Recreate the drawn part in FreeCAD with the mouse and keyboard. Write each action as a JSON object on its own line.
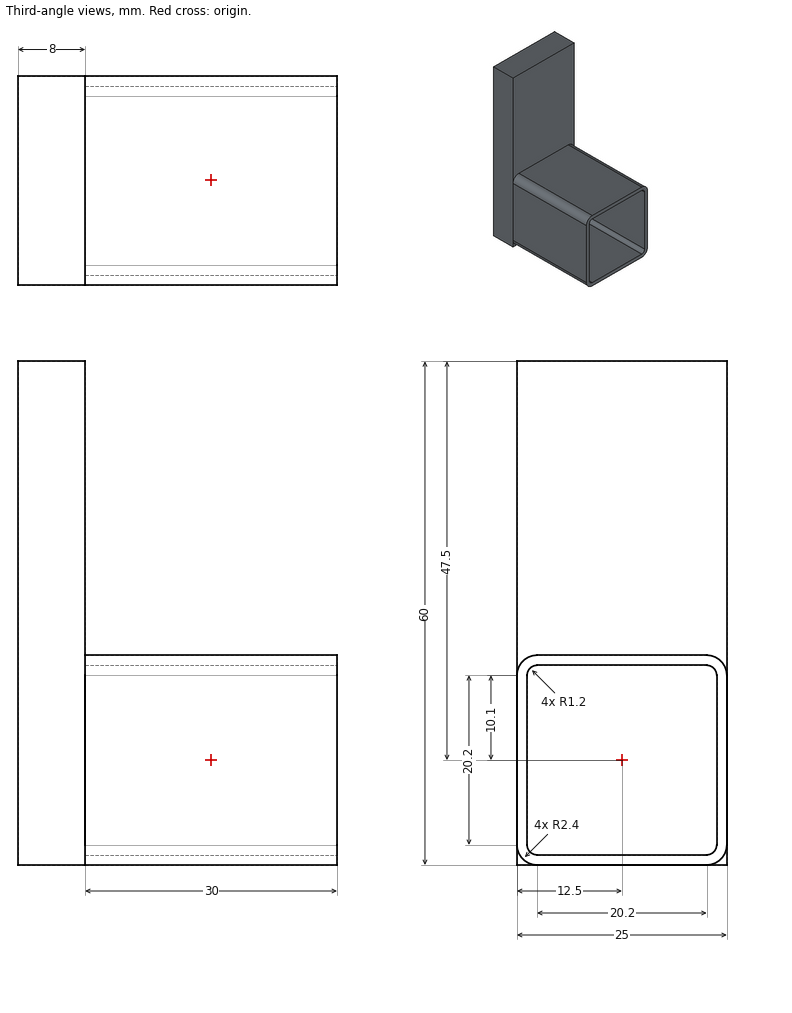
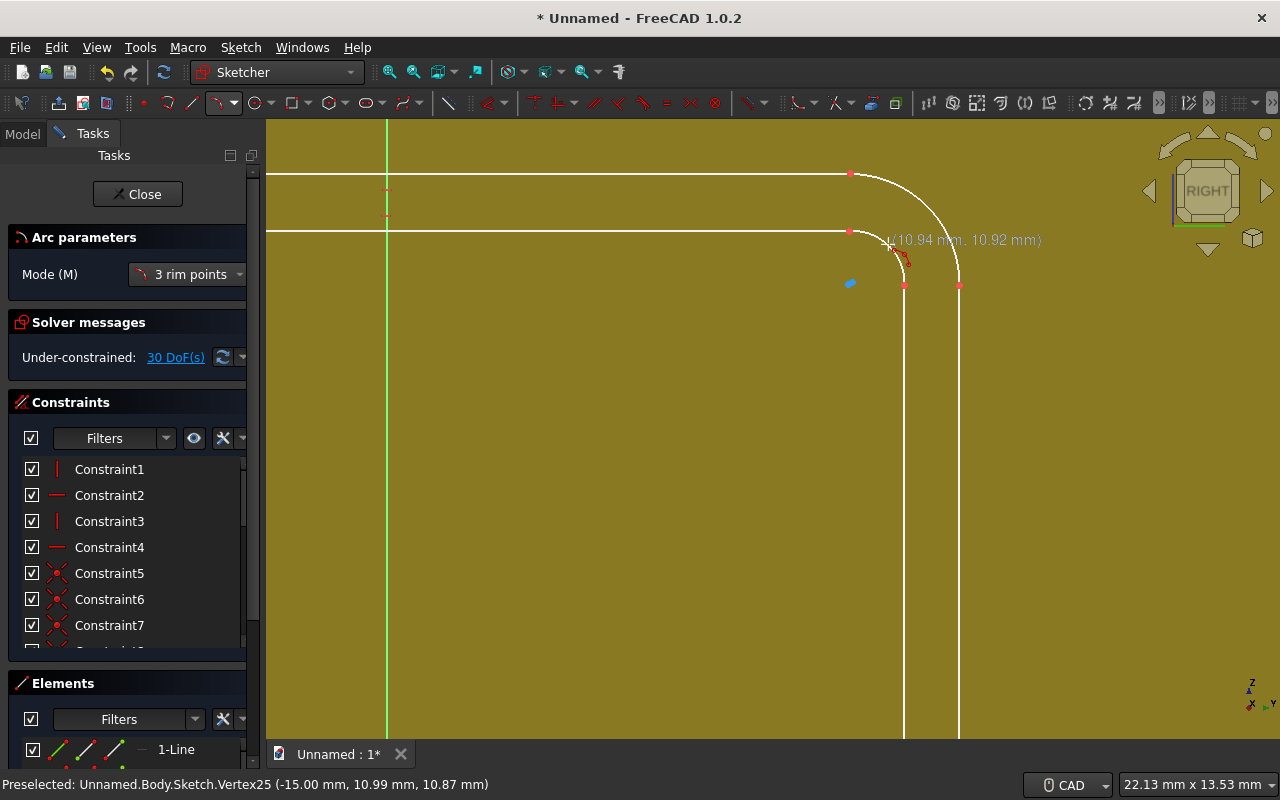
{"action": "scroll", "coordinate": [889, 245], "scroll_direction": "down", "scroll_amount": 5}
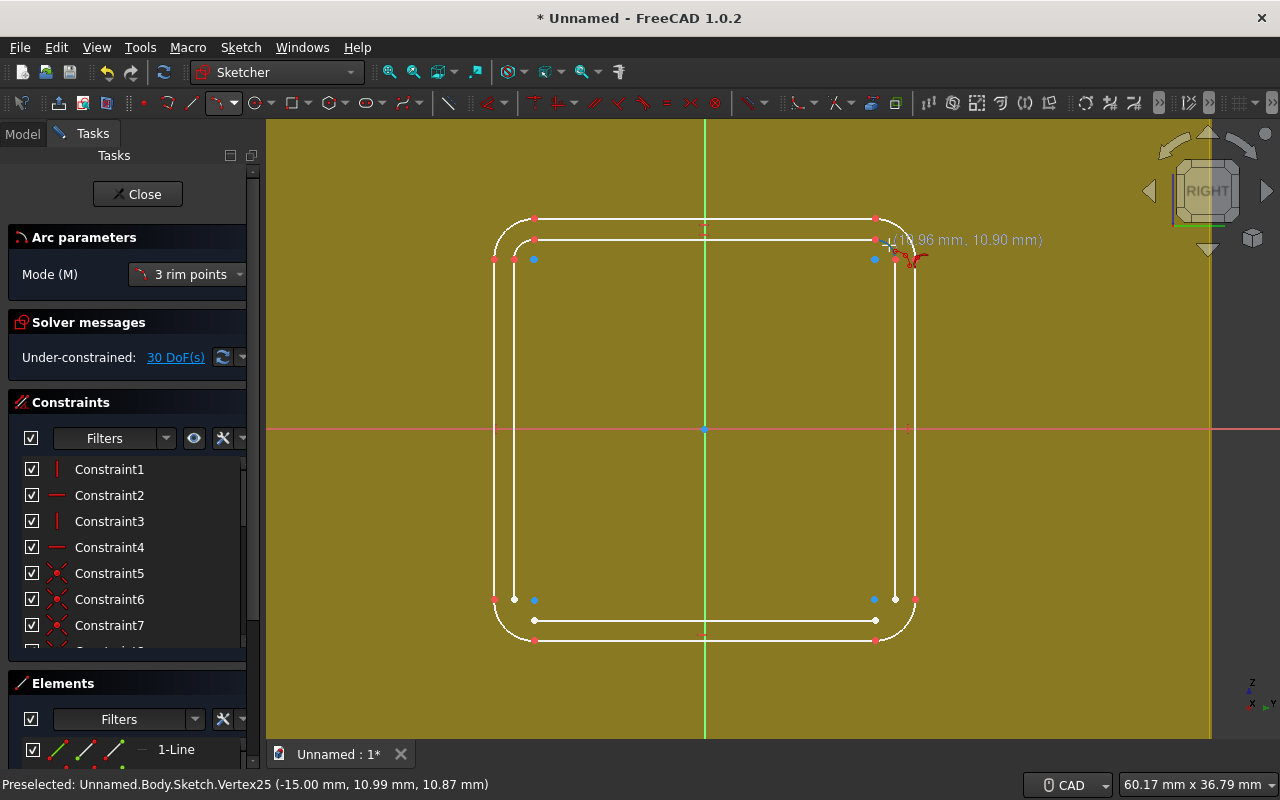
{"action": "left_click", "coordinate": [895, 600]}
{"action": "left_click", "coordinate": [875, 621]}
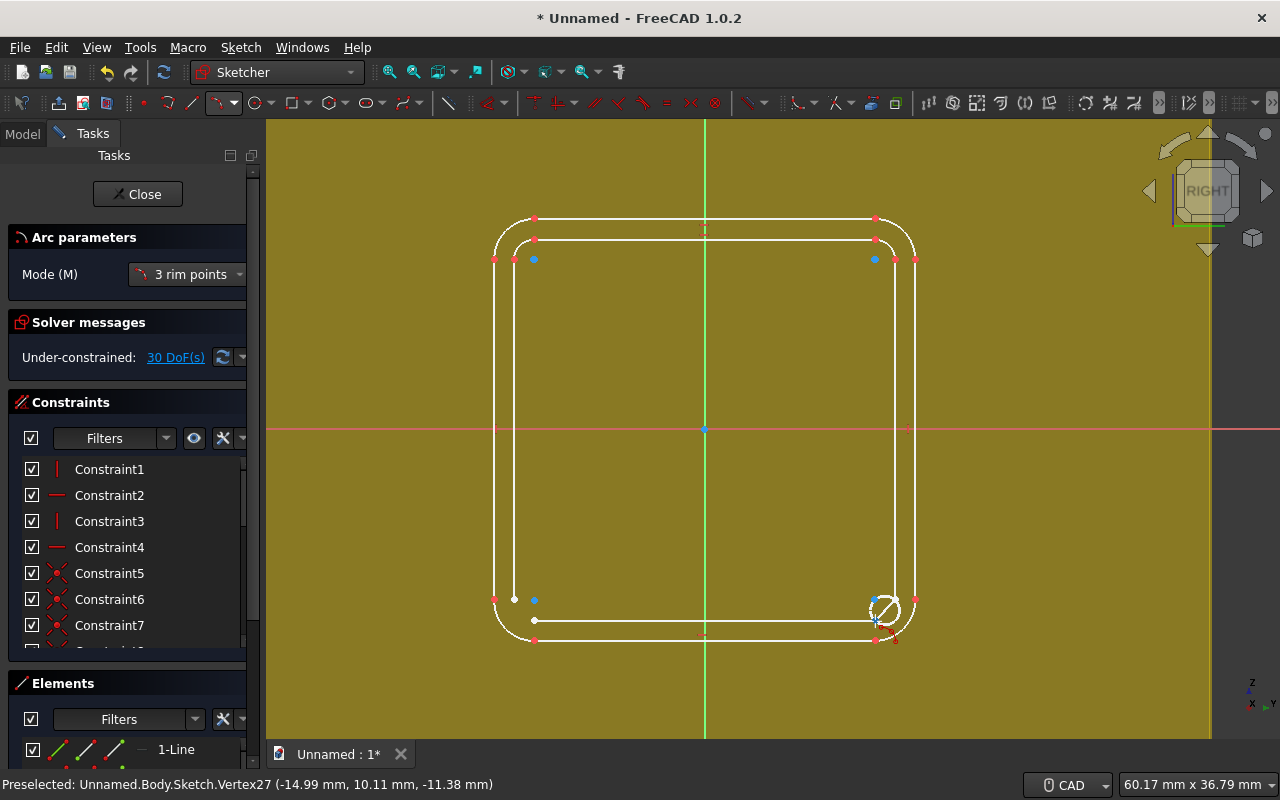
{"action": "scroll", "coordinate": [889, 614], "scroll_direction": "up", "scroll_amount": 5}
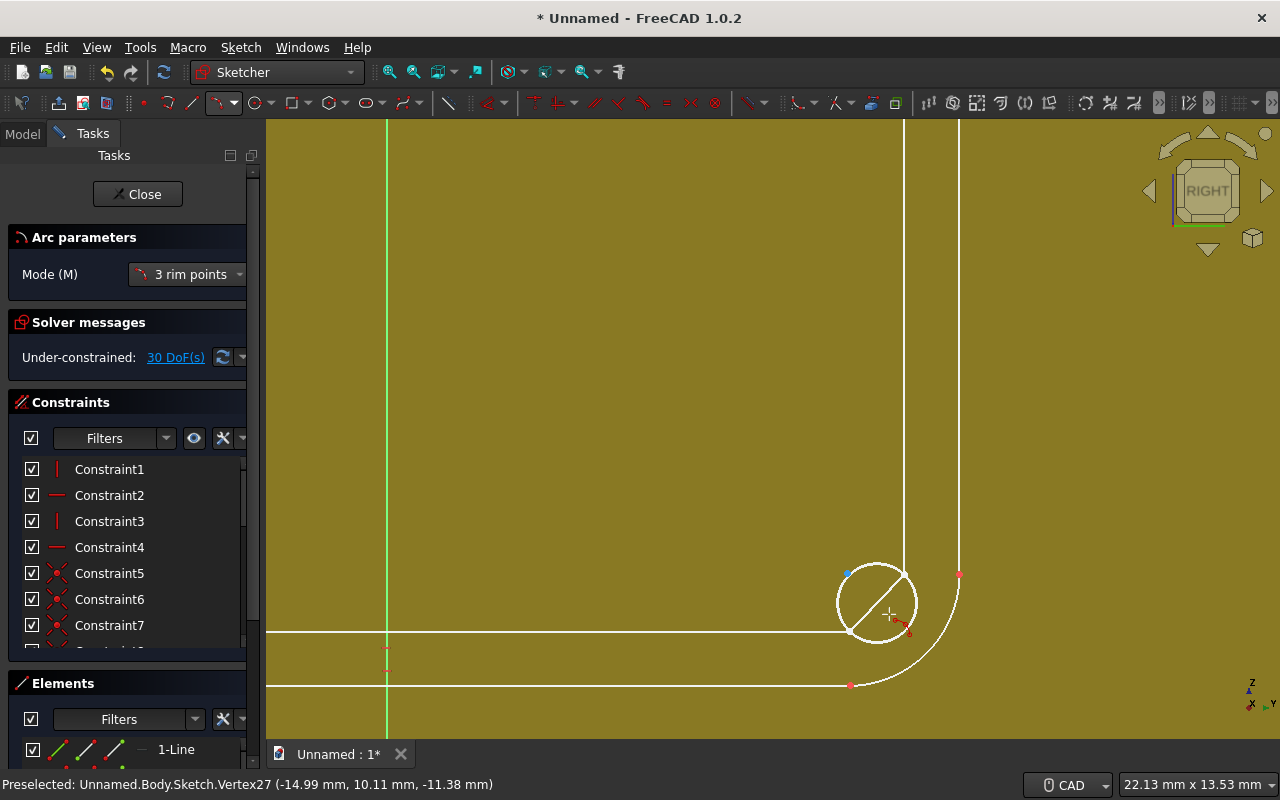
{"action": "left_click", "coordinate": [888, 612]}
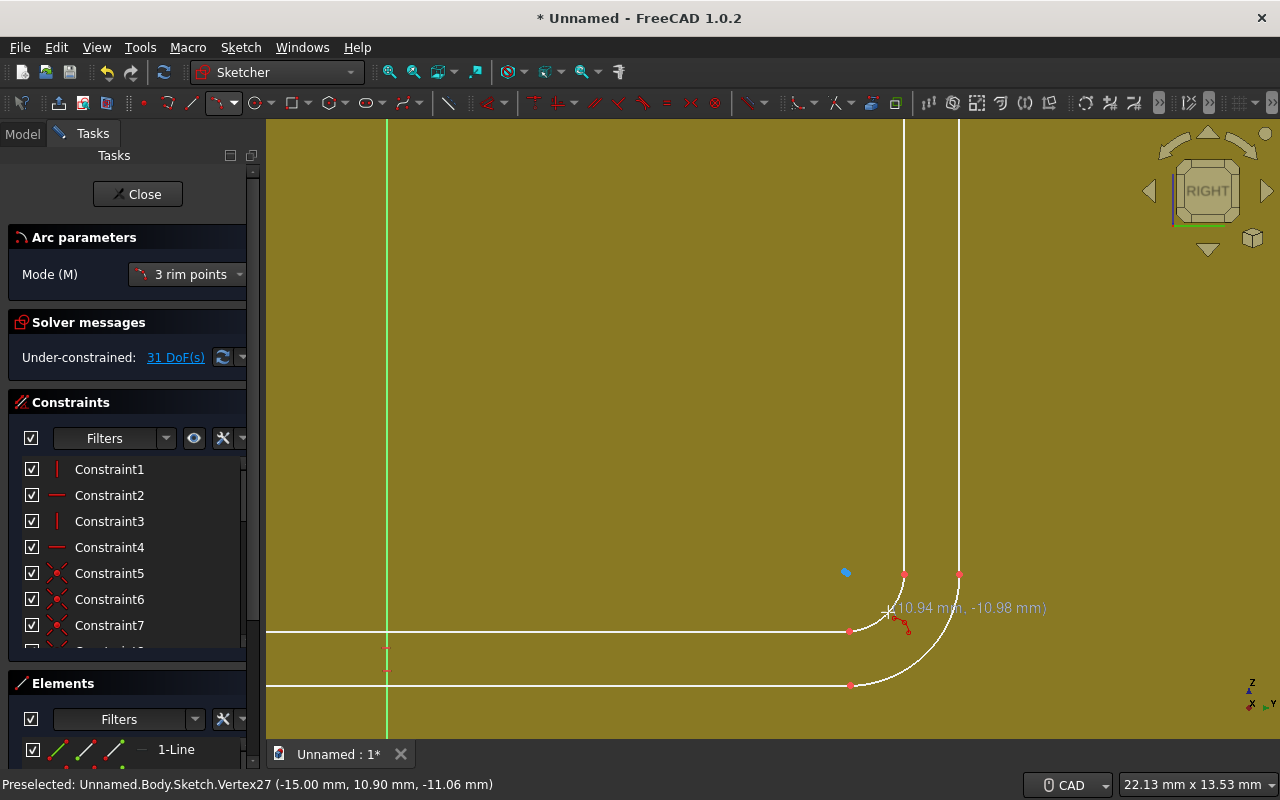
{"action": "scroll", "coordinate": [889, 615], "scroll_direction": "down", "scroll_amount": 5}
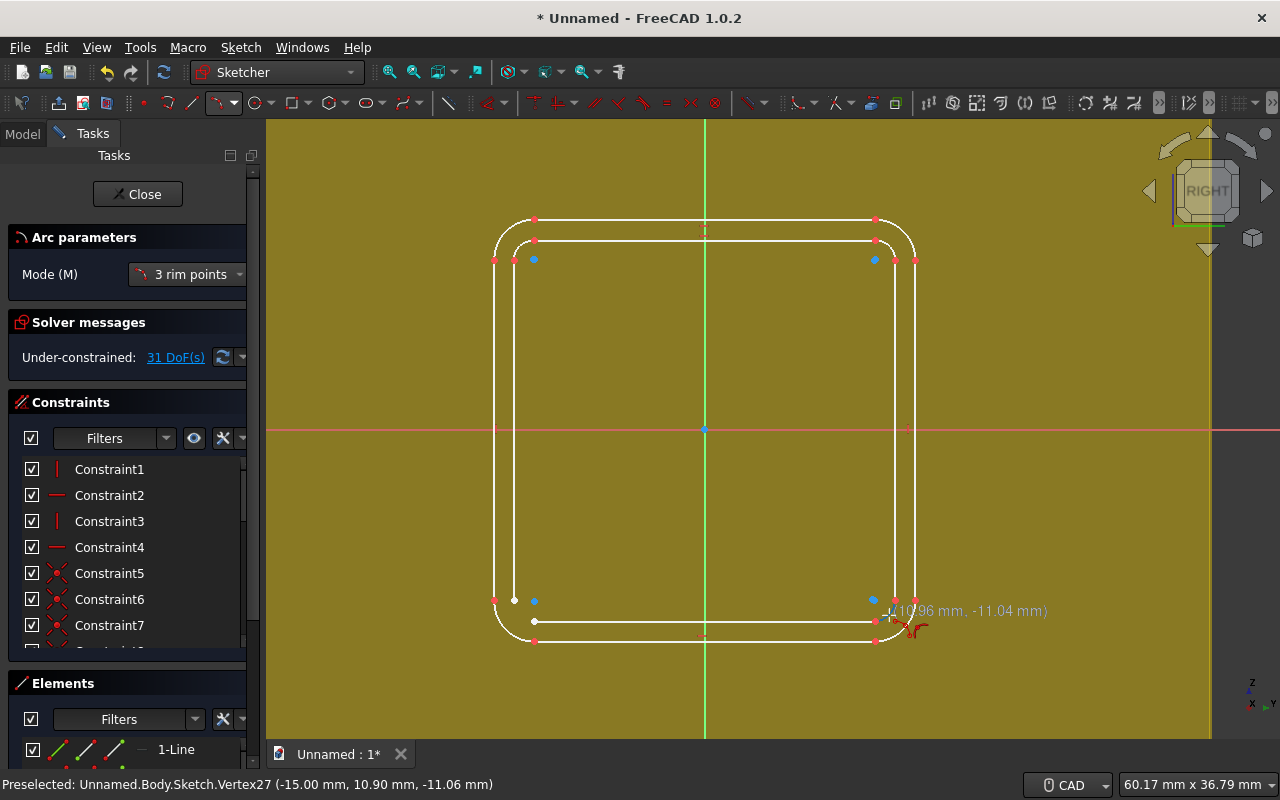
{"action": "left_click", "coordinate": [534, 622]}
{"action": "left_click", "coordinate": [514, 601]}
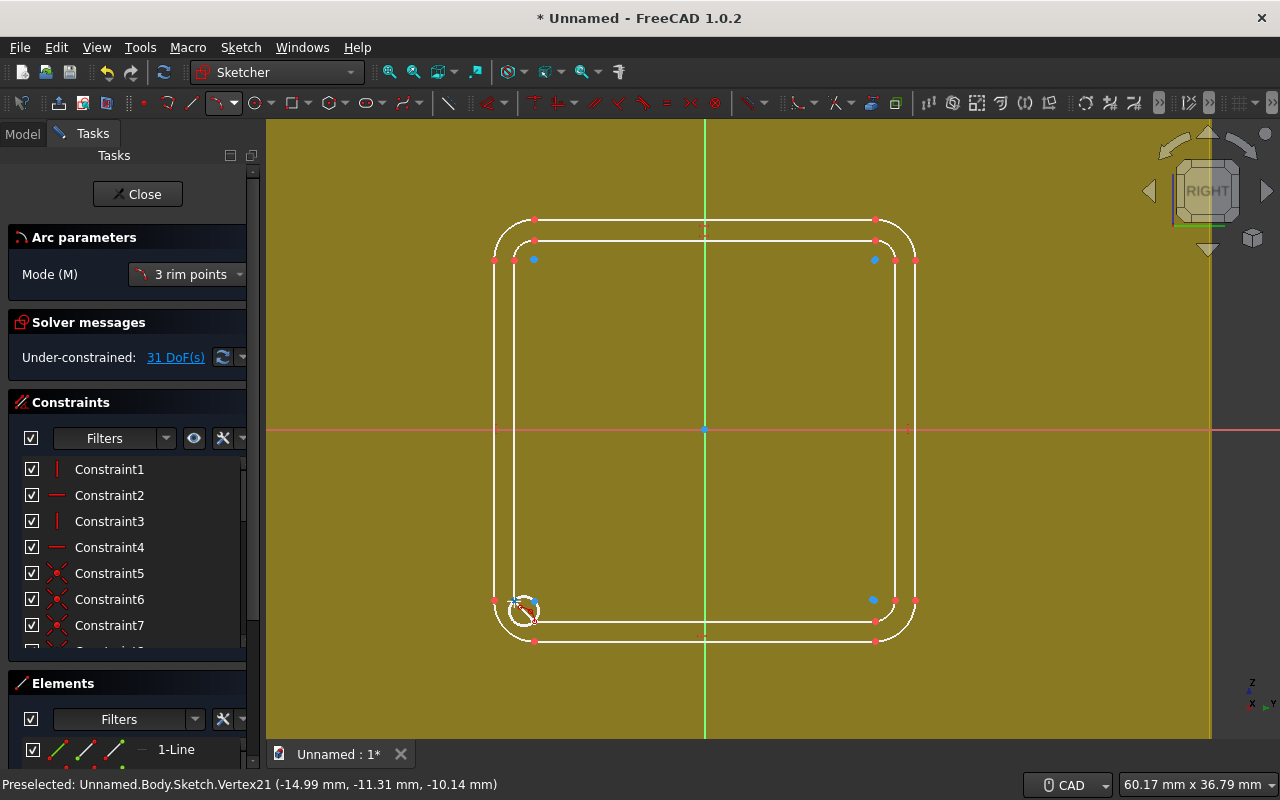
{"action": "scroll", "coordinate": [520, 614], "scroll_direction": "up", "scroll_amount": 5}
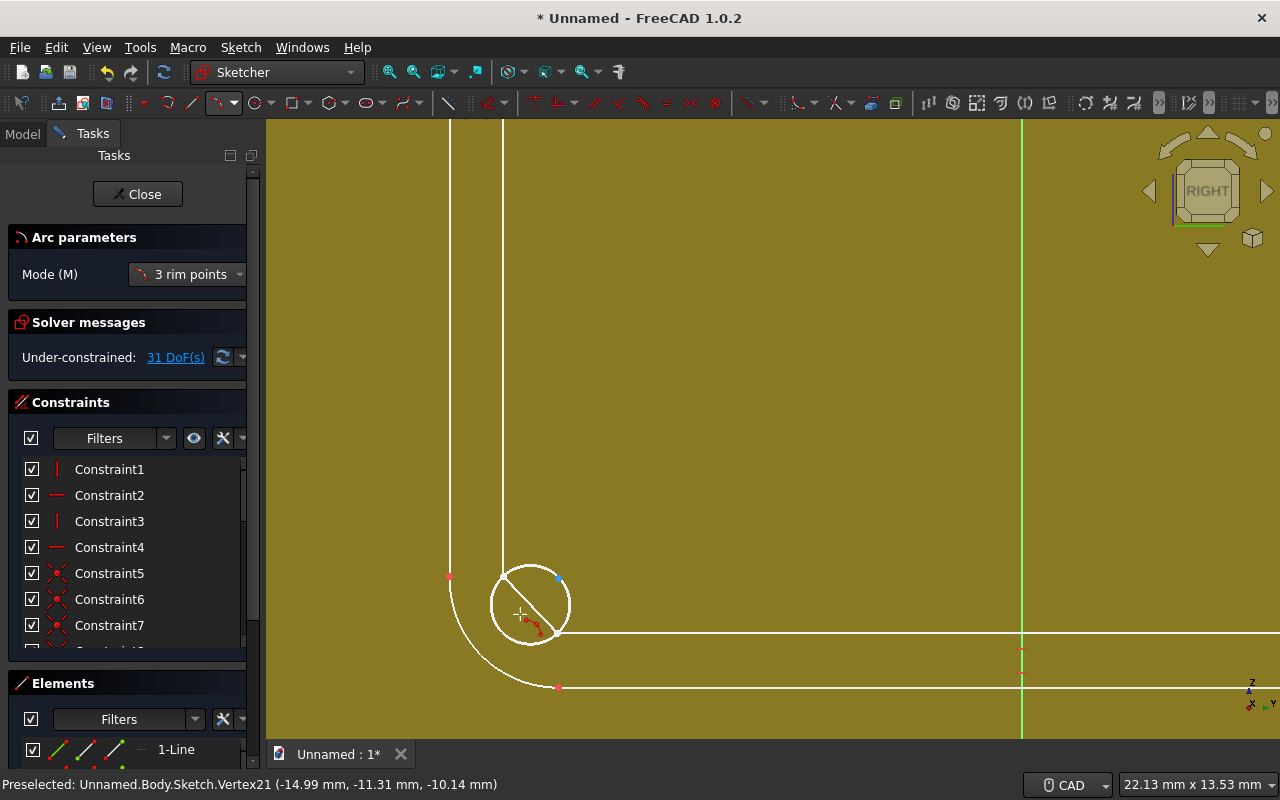
{"action": "left_click", "coordinate": [520, 613]}
{"action": "key", "text": "Escape"}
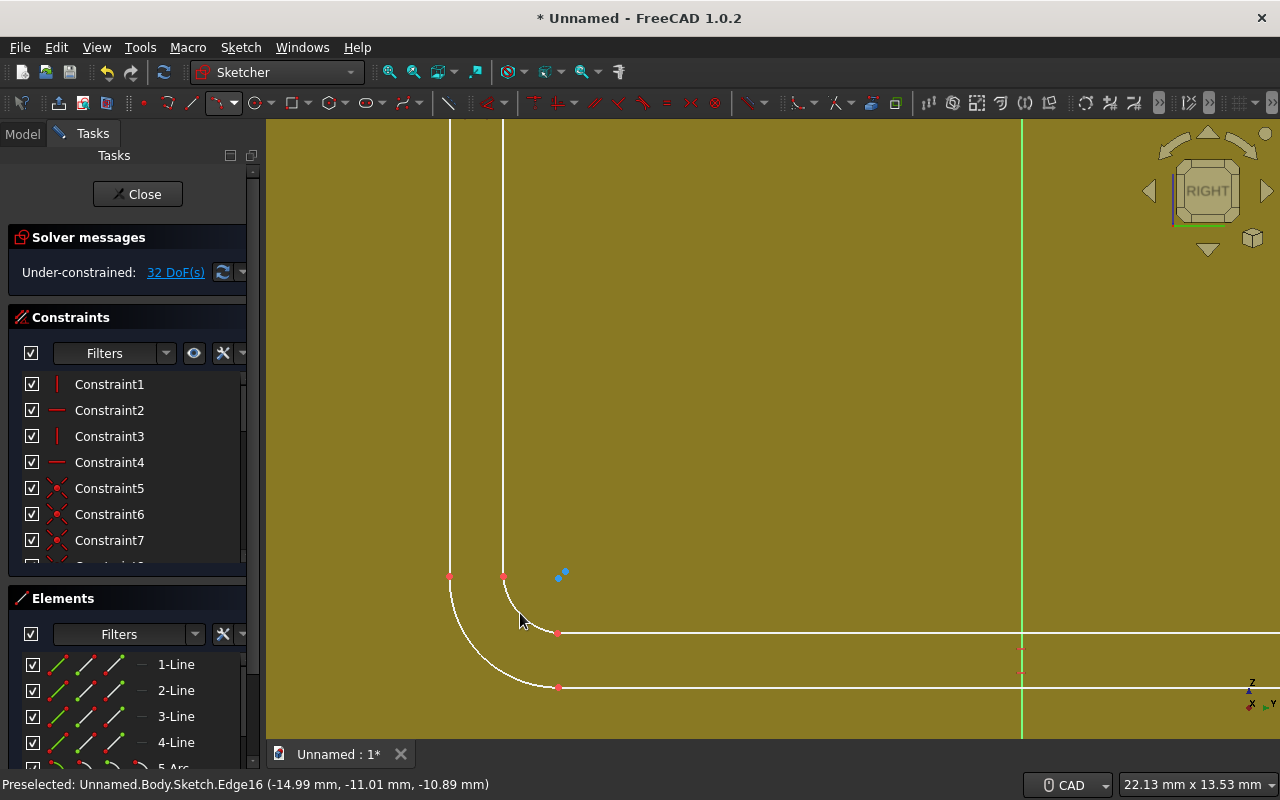
{"action": "left_click", "coordinate": [450, 299]}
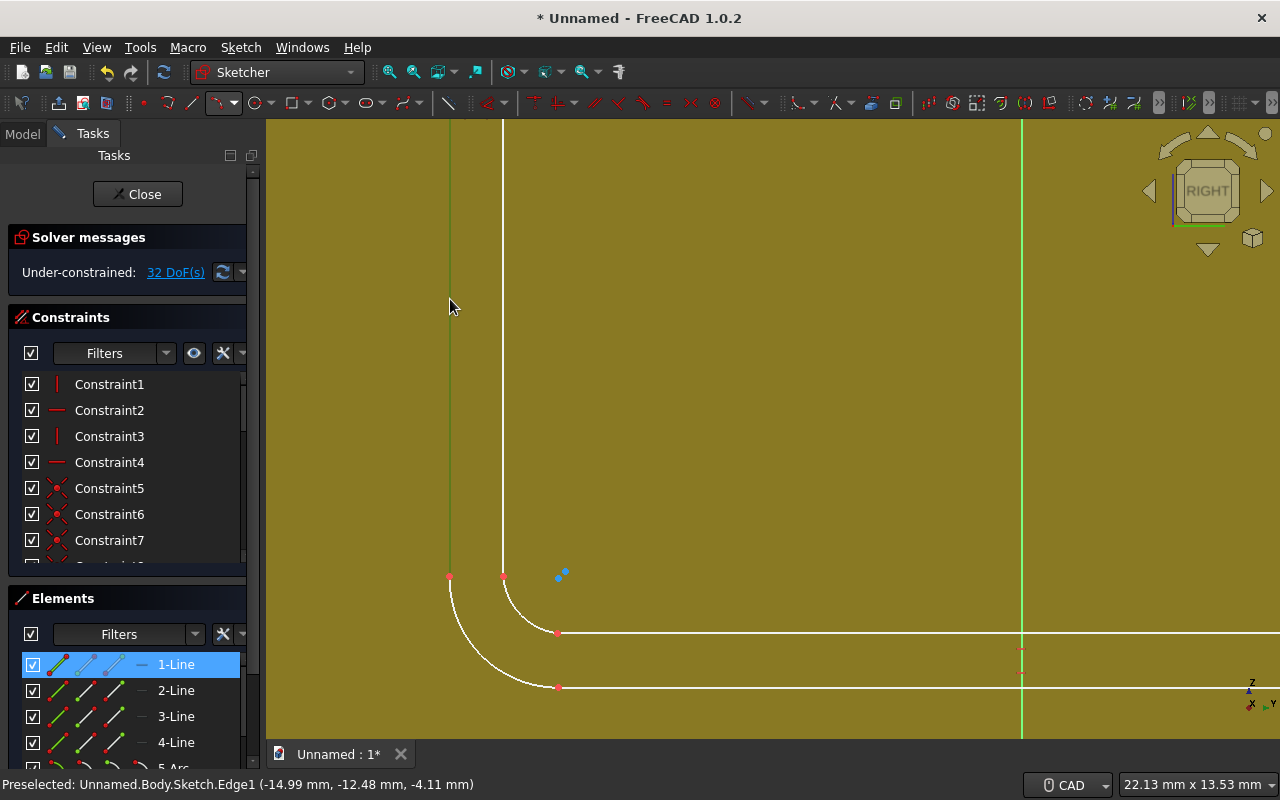
{"action": "left_click", "coordinate": [461, 627]}